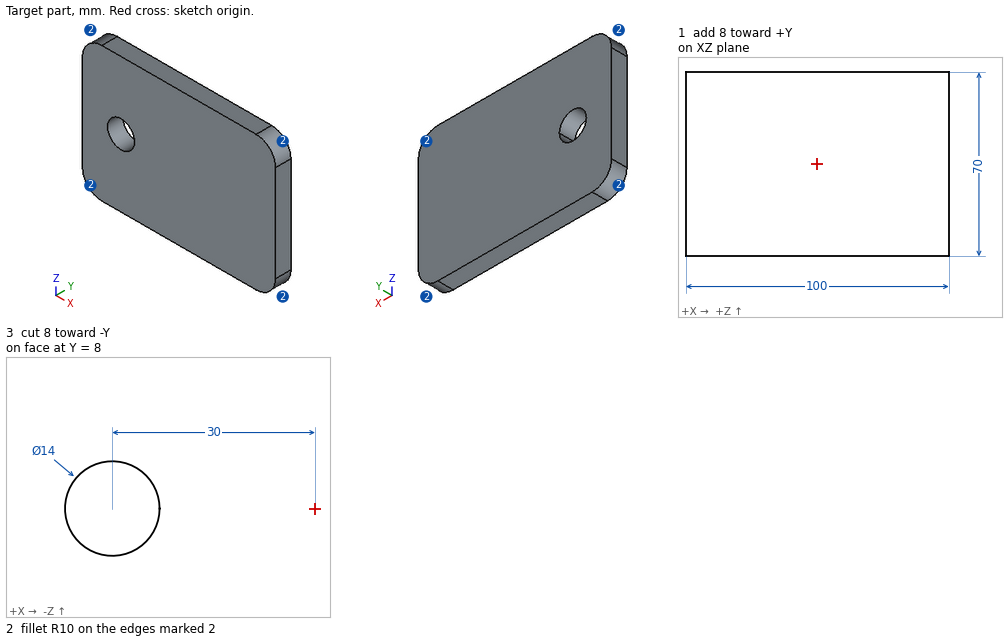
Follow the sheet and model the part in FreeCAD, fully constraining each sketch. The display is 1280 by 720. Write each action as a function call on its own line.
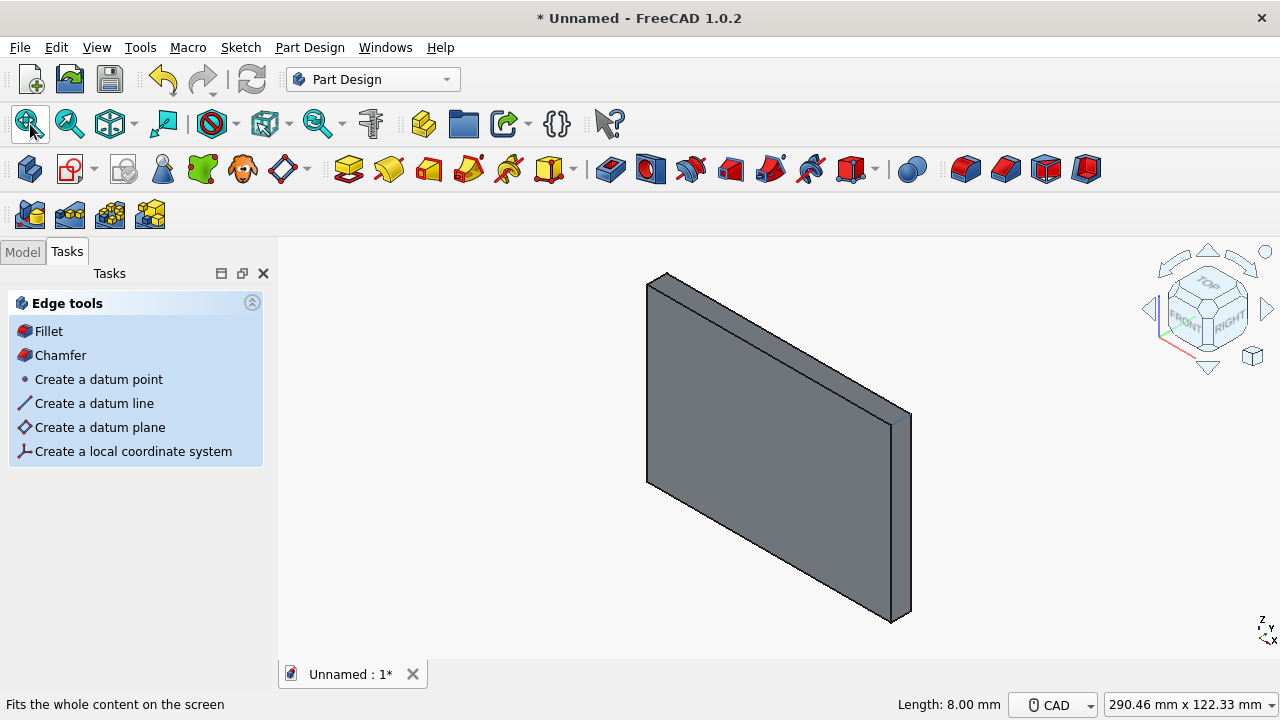
key(2)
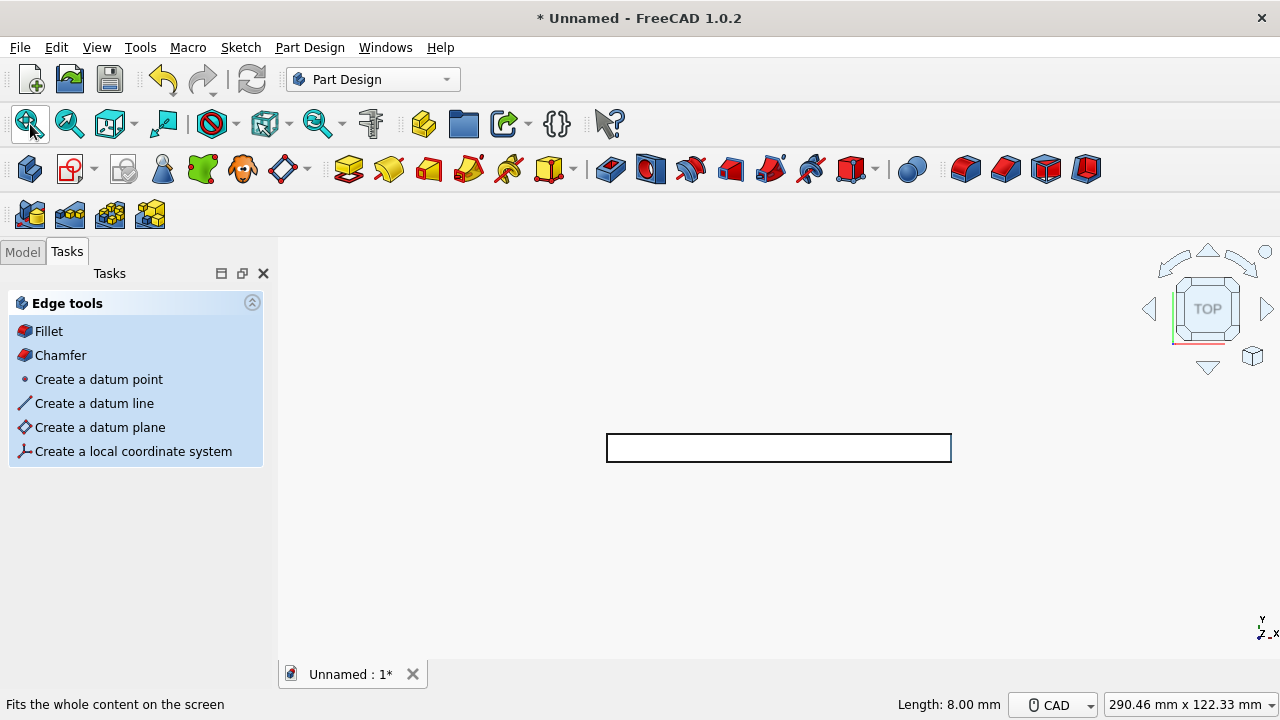
click(30, 124)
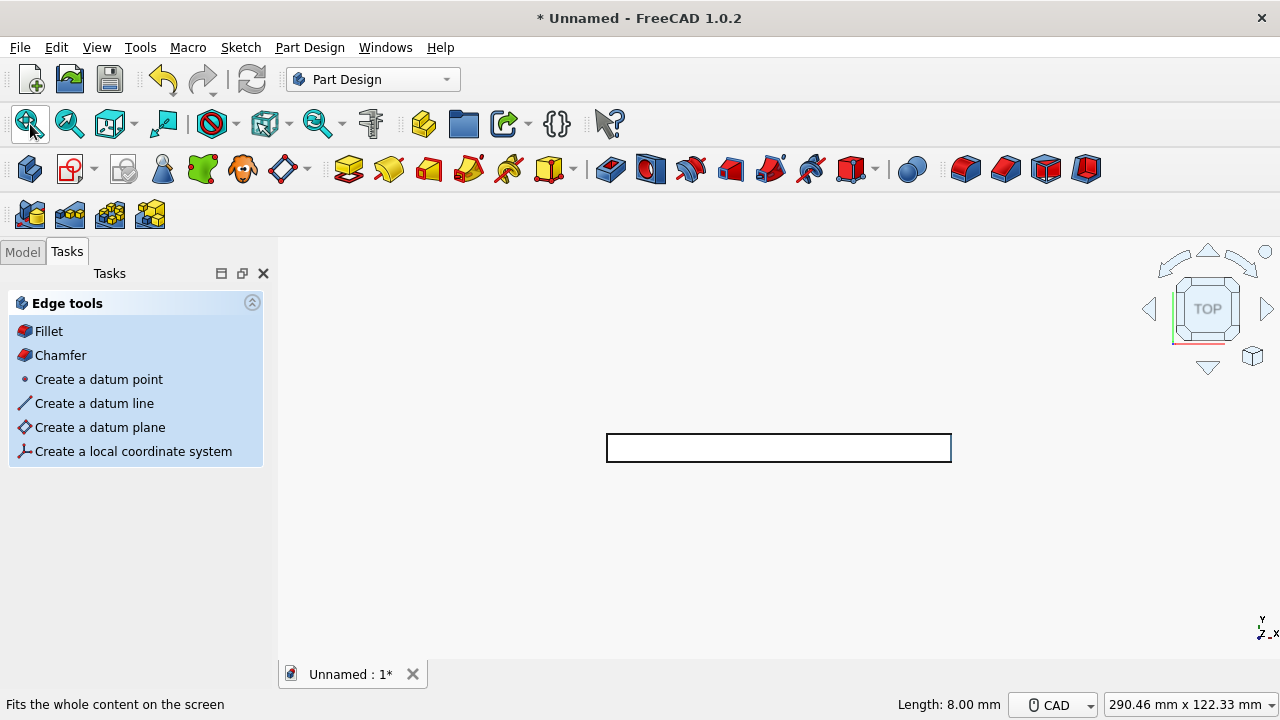
click(607, 447, ctrl)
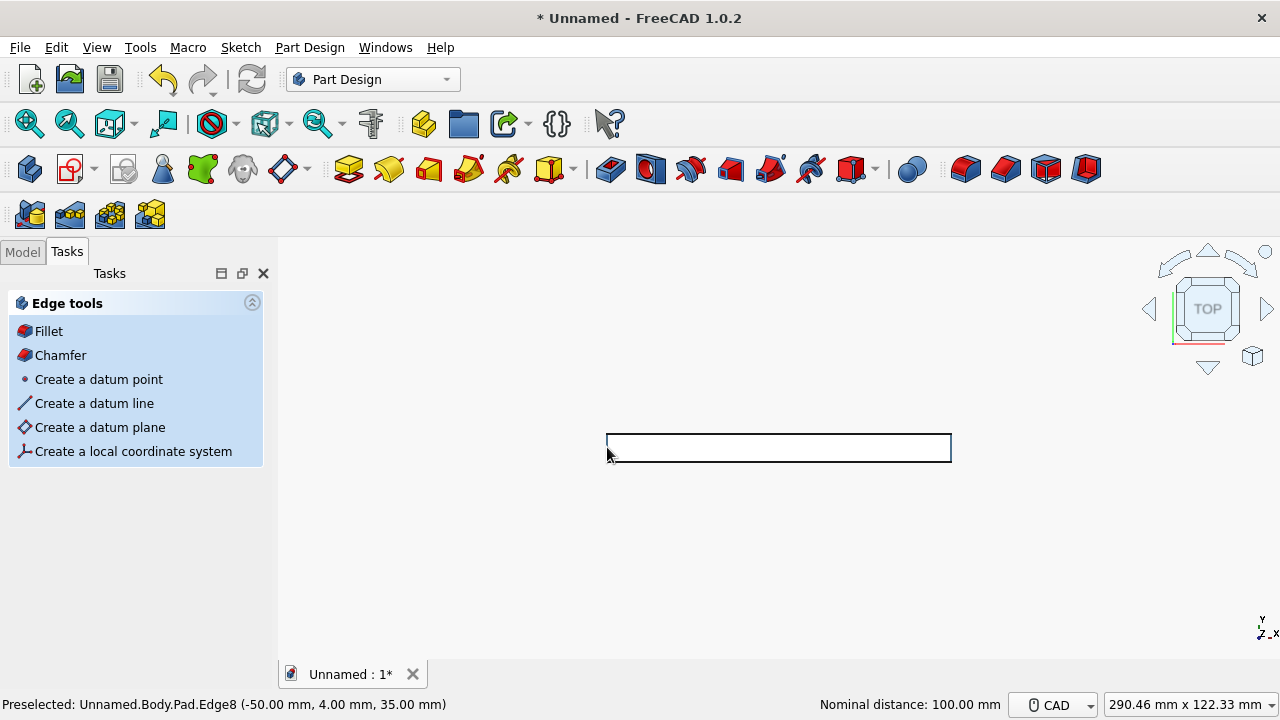
key(1)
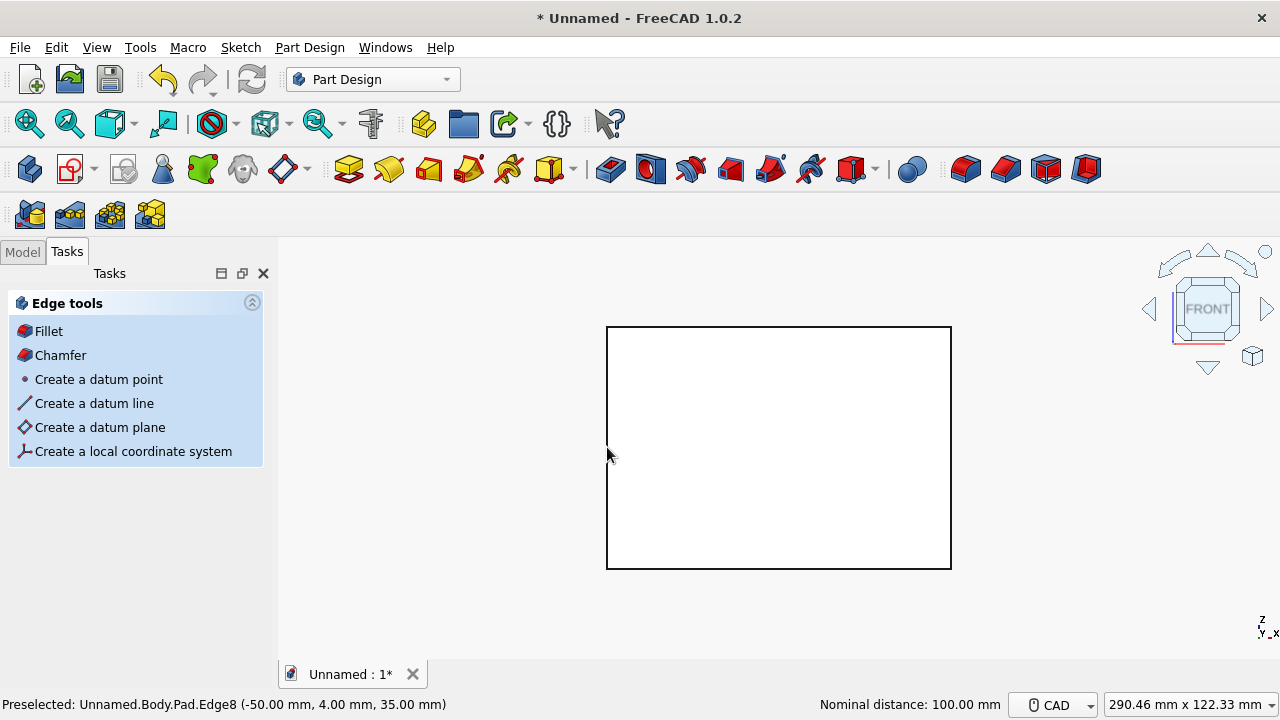
key(3)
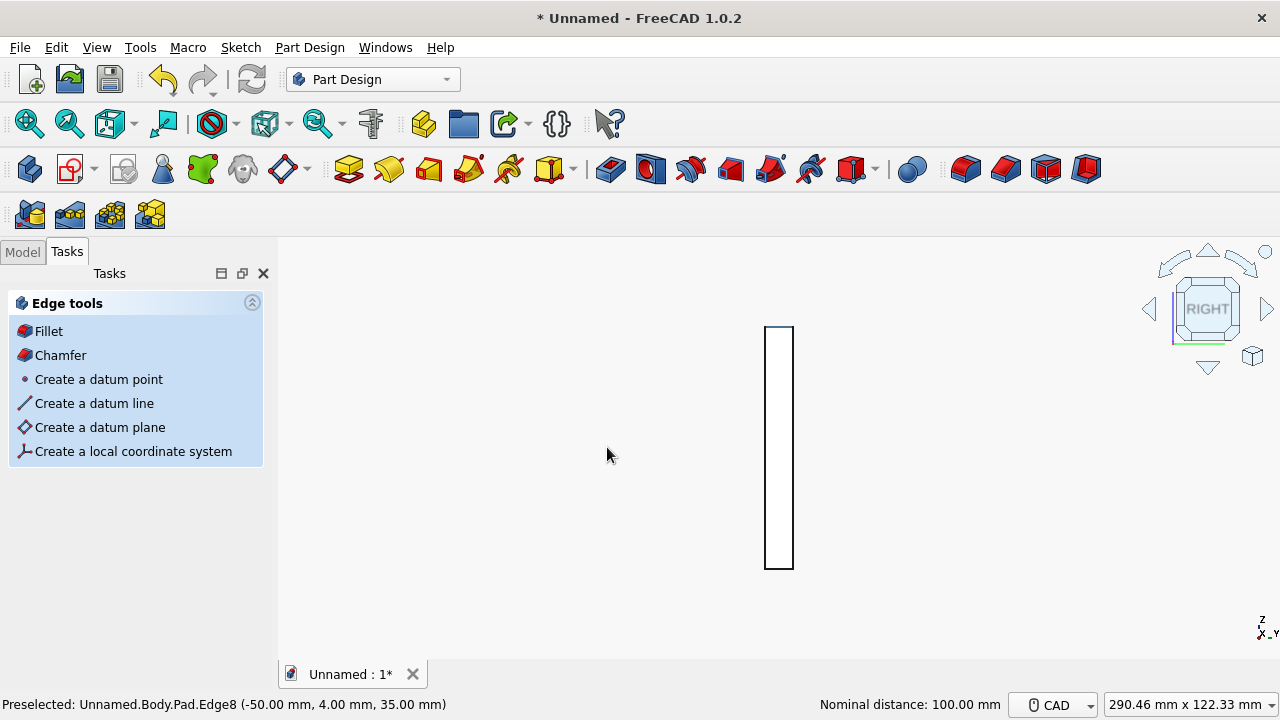
click(779, 568, ctrl)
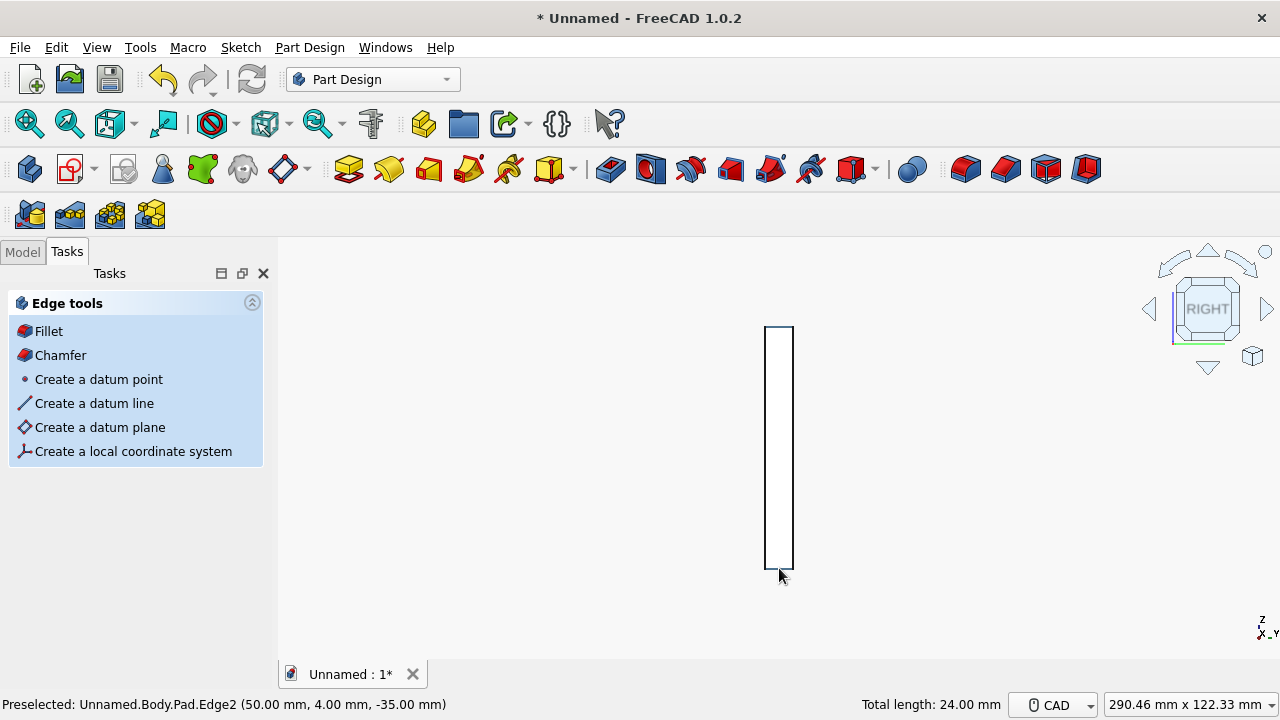
key(5)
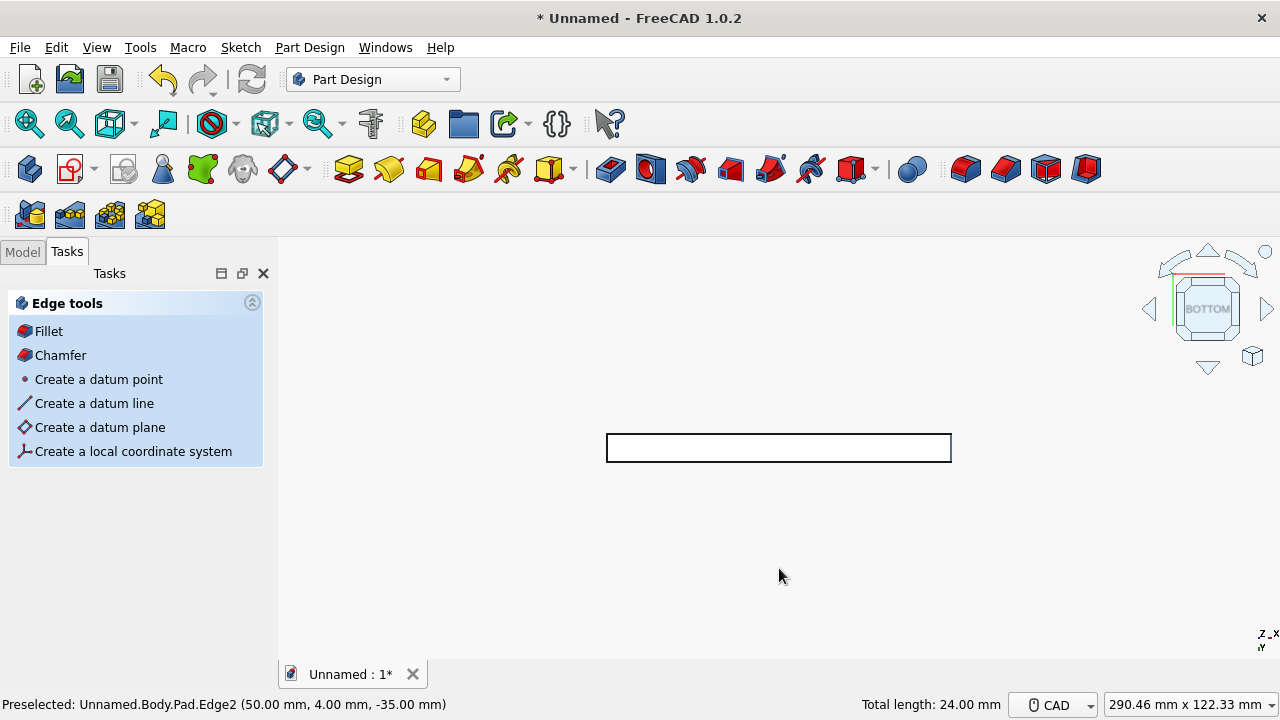
click(30, 124)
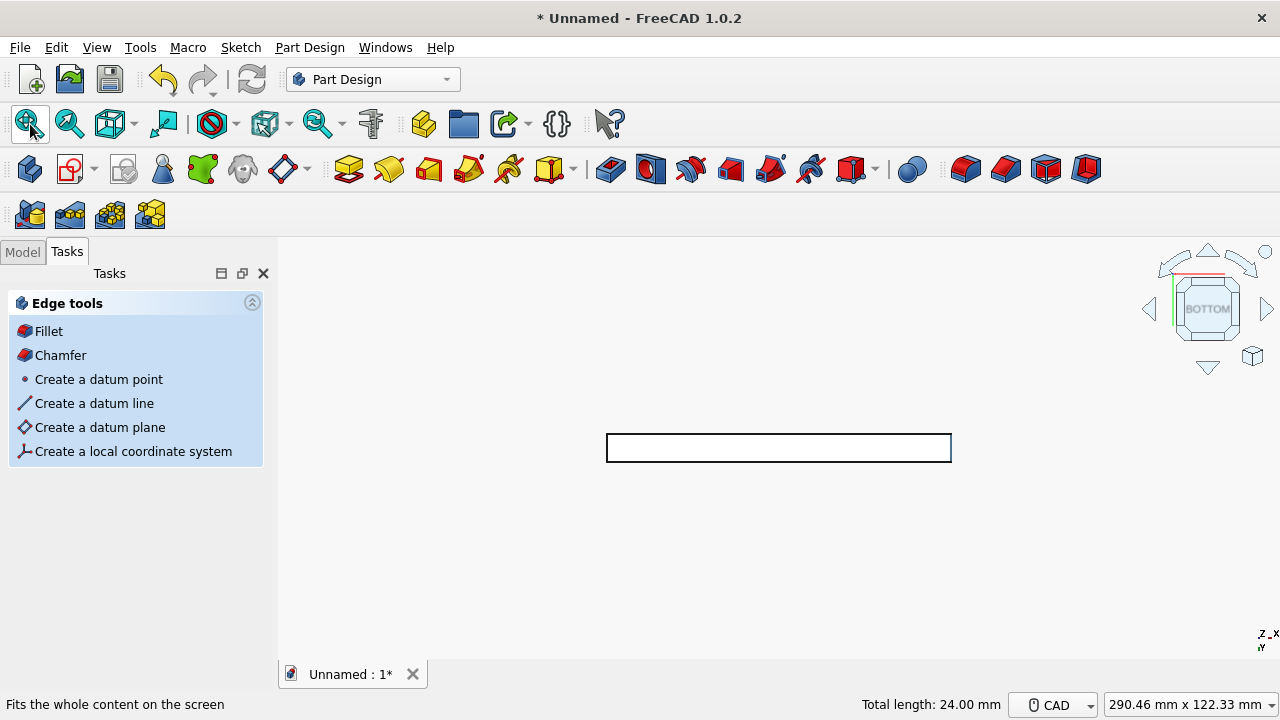
click(607, 447, ctrl)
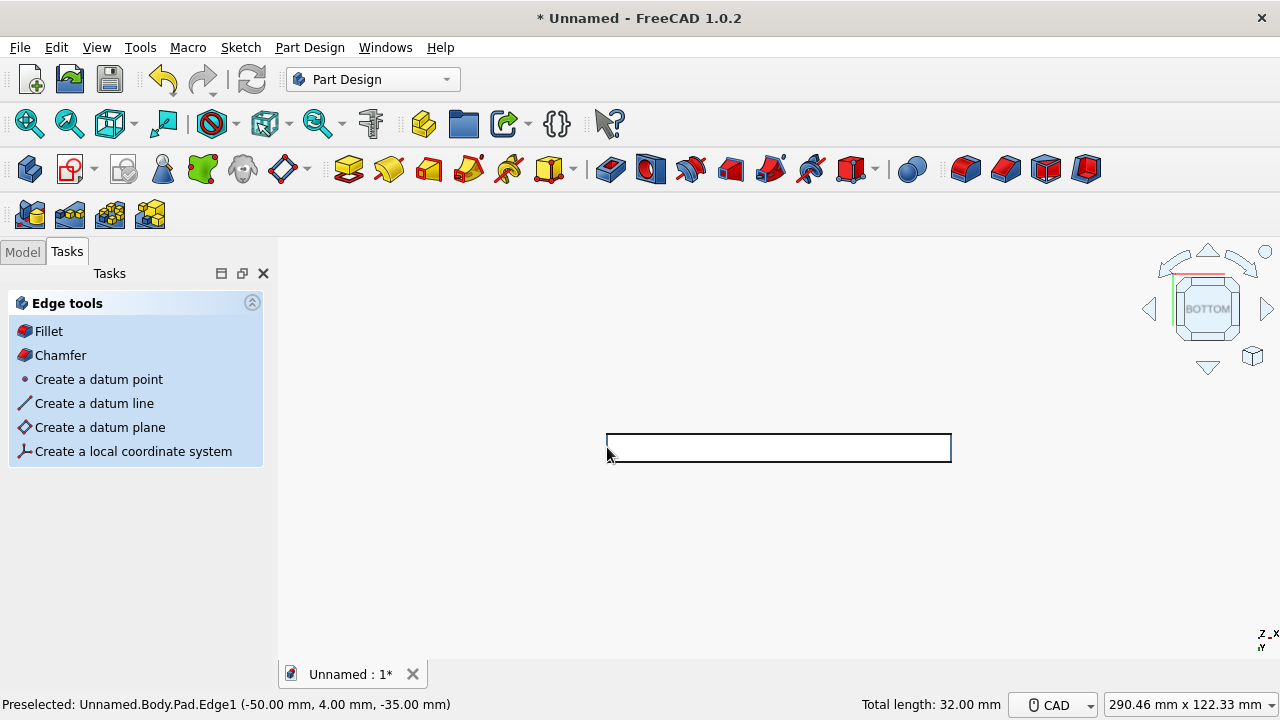
click(966, 170)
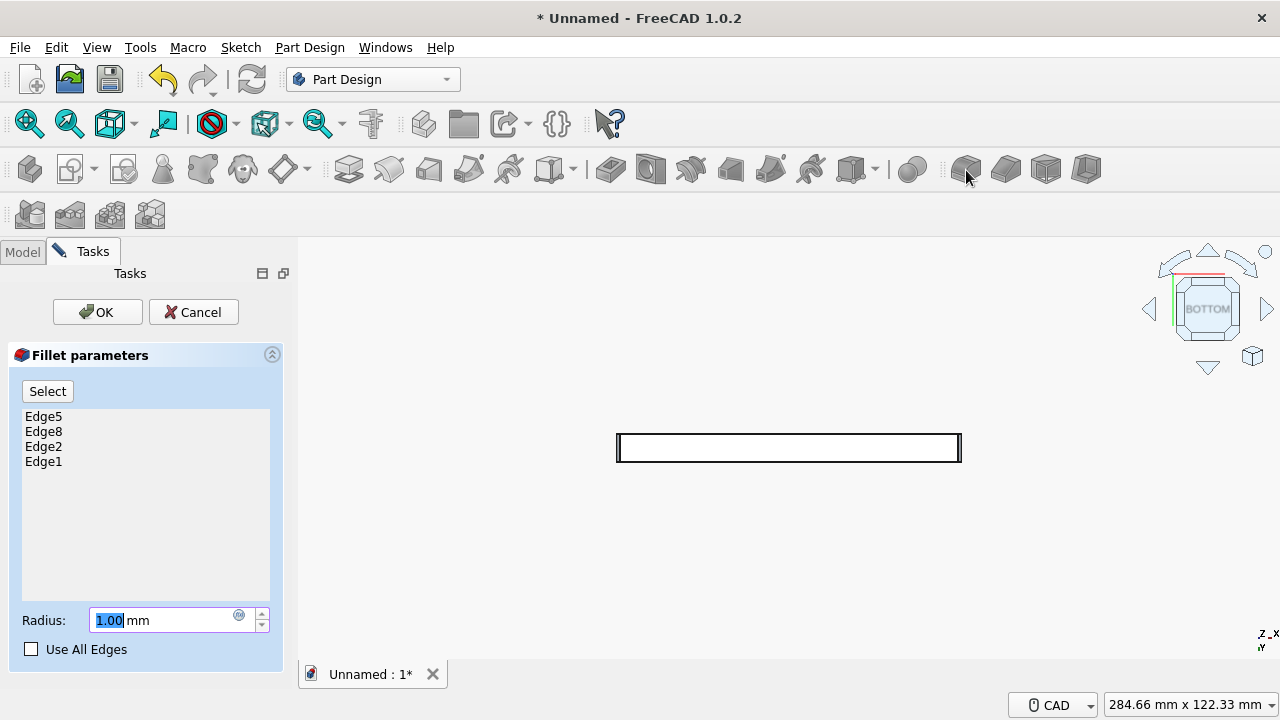
text(10)
key(Tab)